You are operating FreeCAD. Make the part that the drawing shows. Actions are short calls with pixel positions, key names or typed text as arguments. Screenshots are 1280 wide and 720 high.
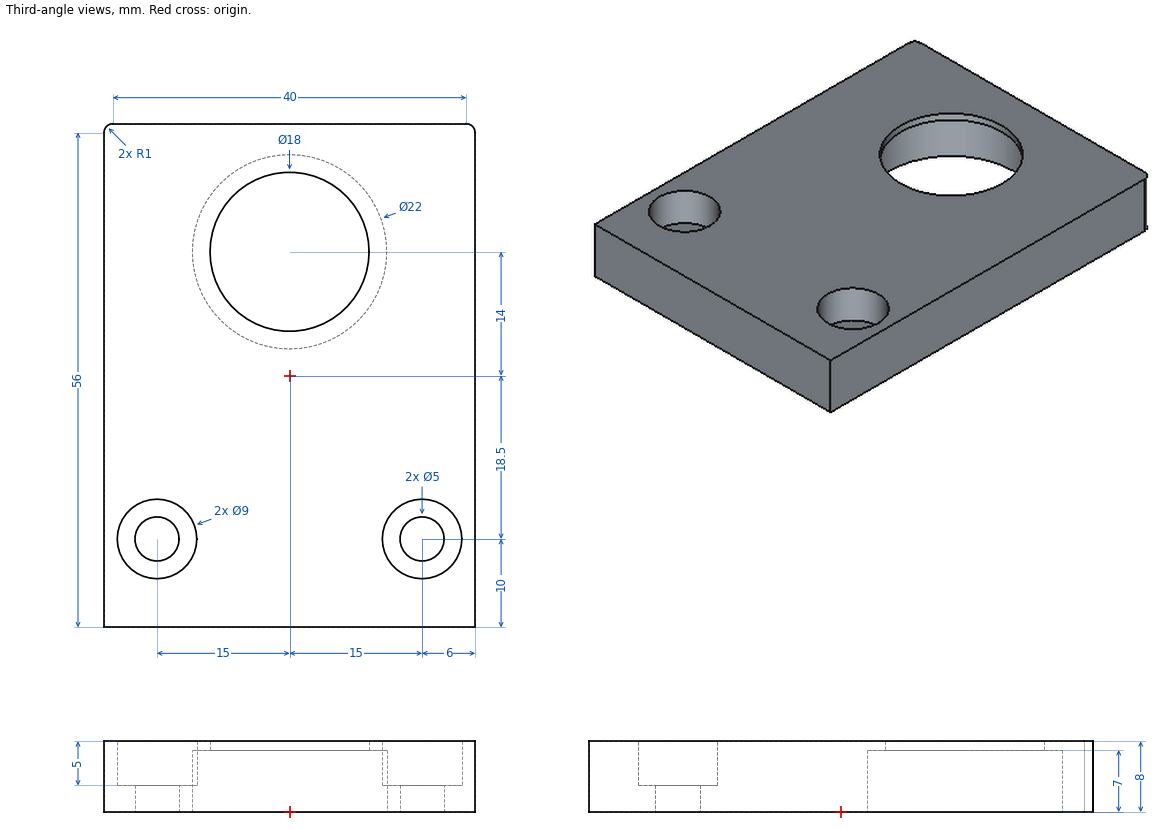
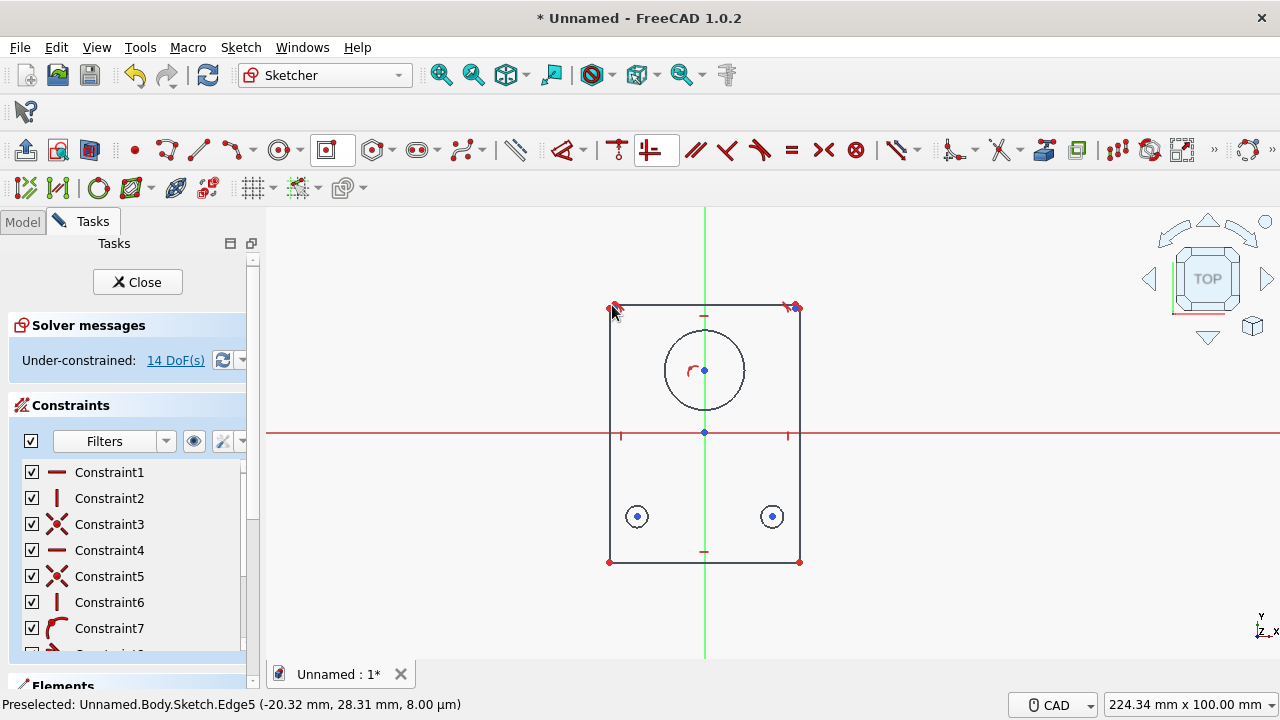
scroll(799, 307, up, 10)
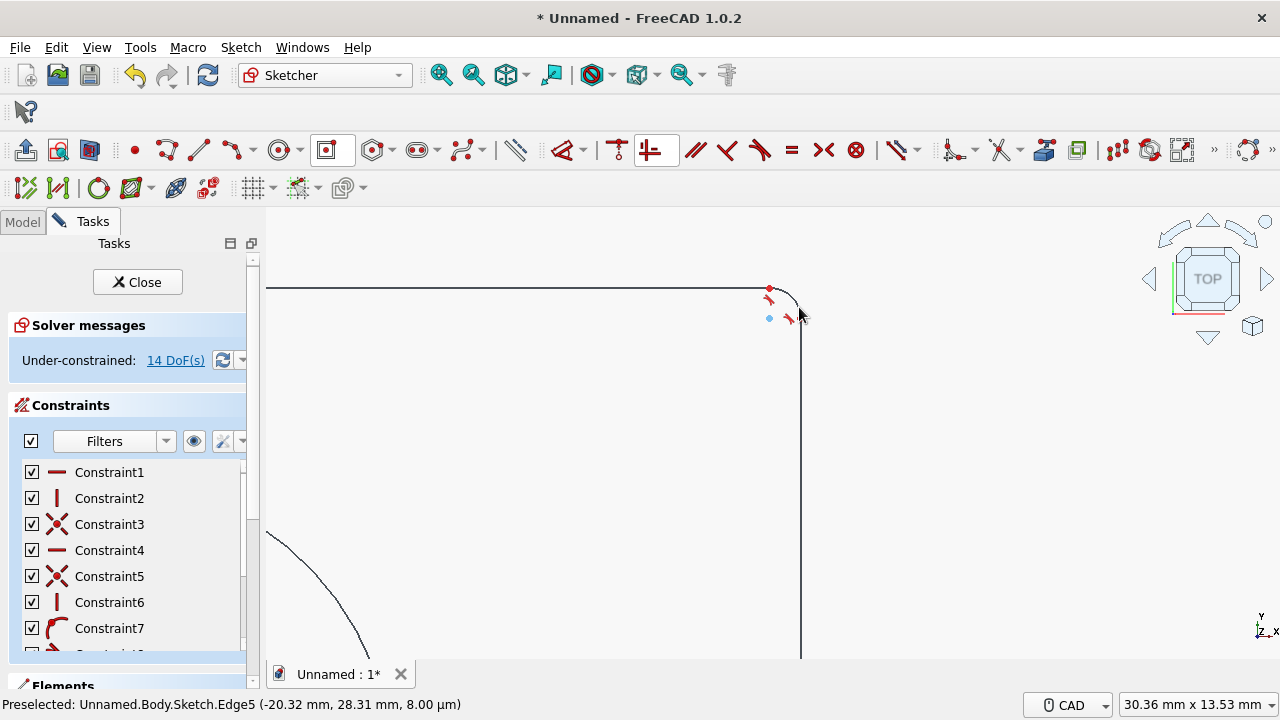
click(798, 305)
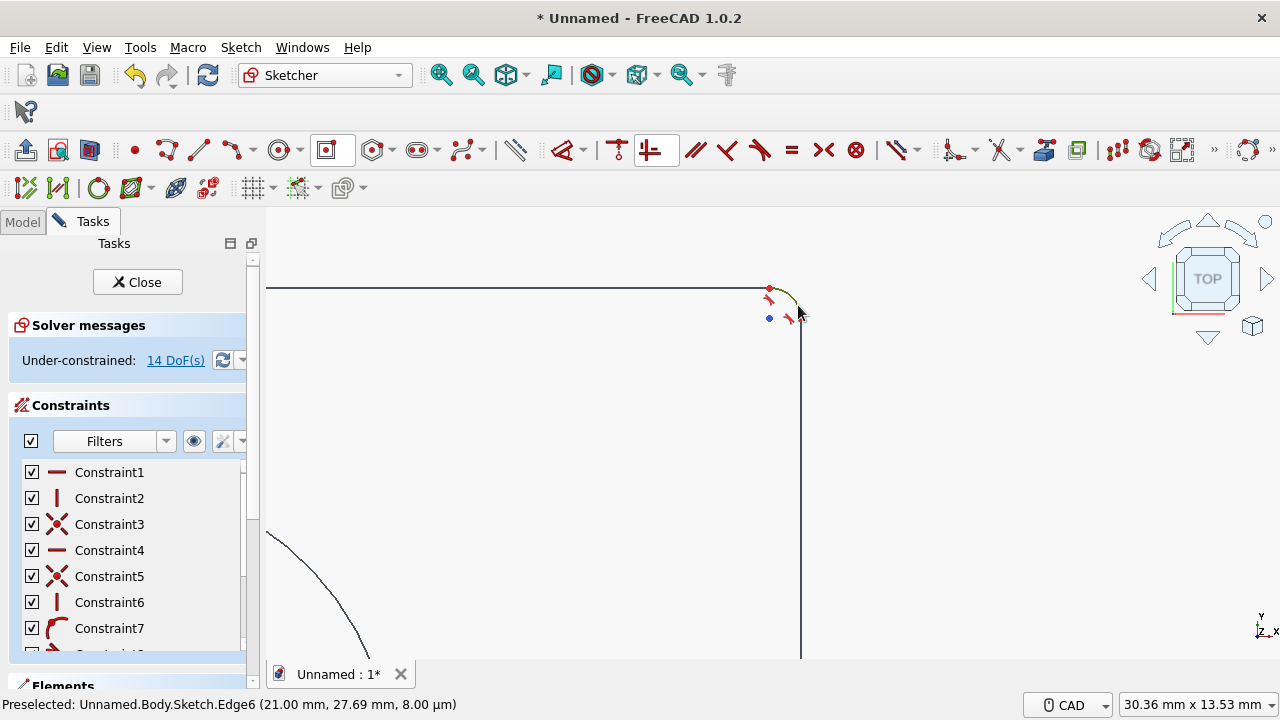
click(792, 150)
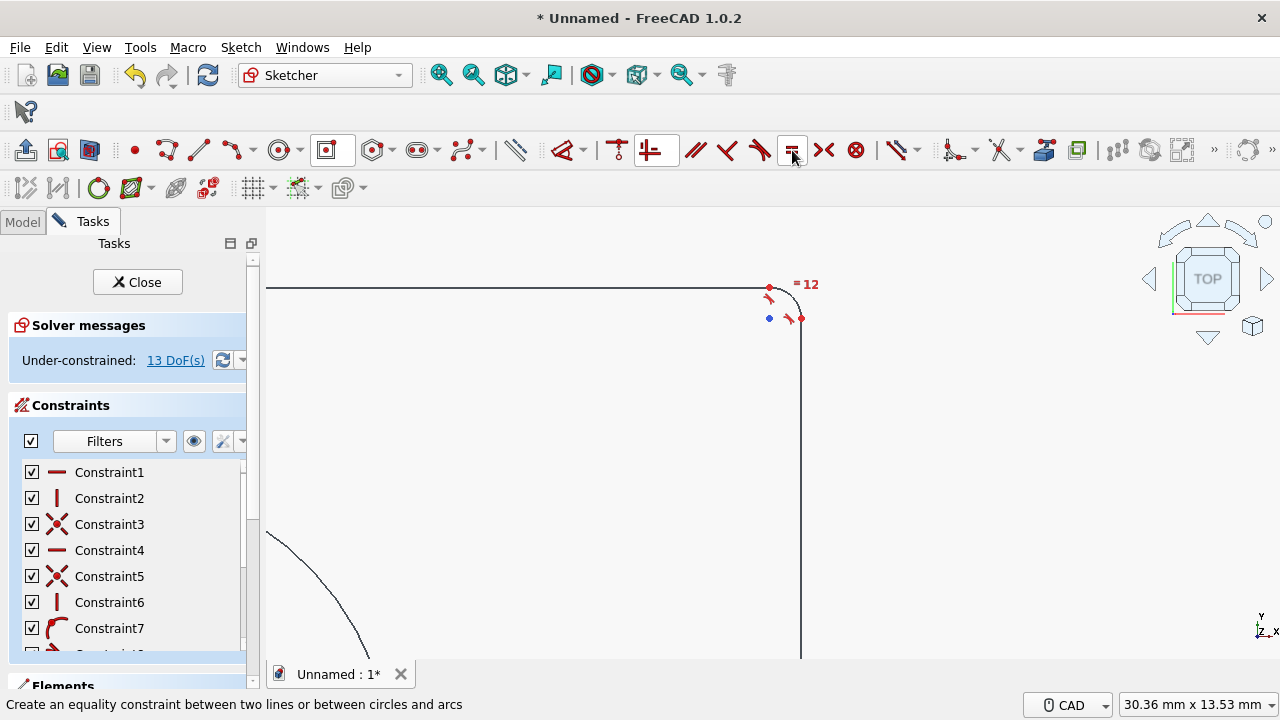
scroll(799, 307, down, 10)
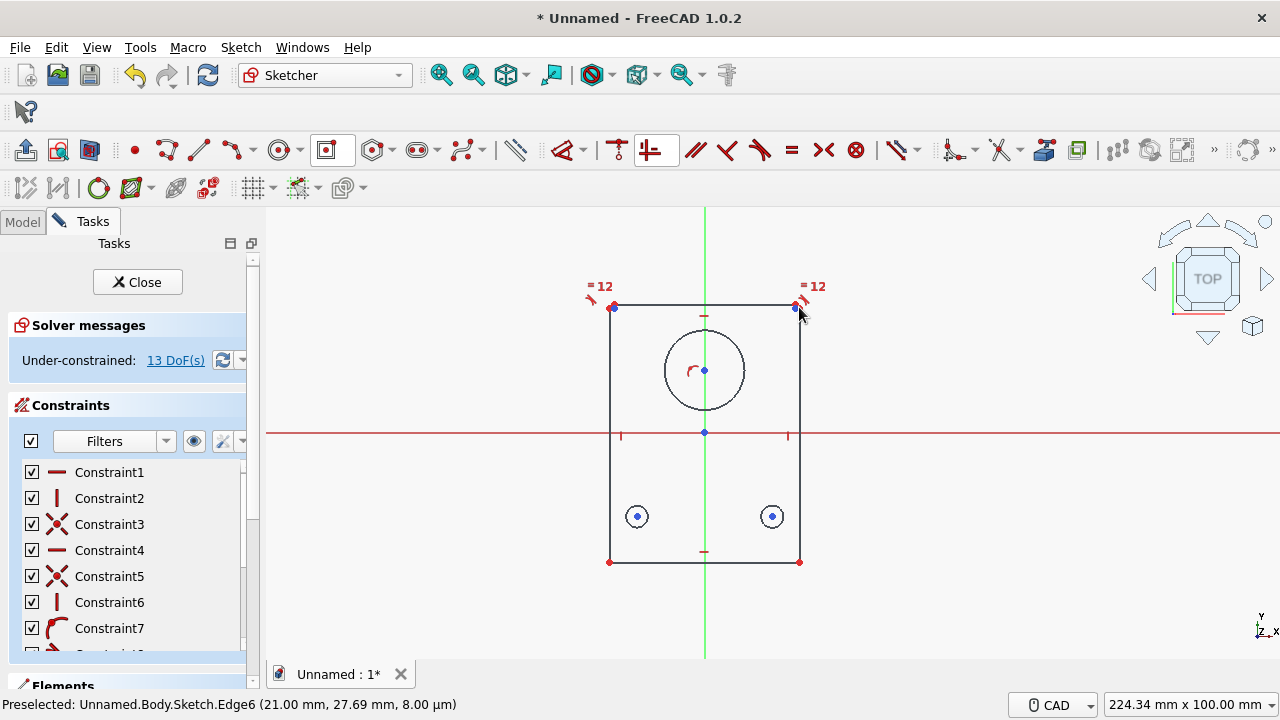
scroll(780, 509, up, 2)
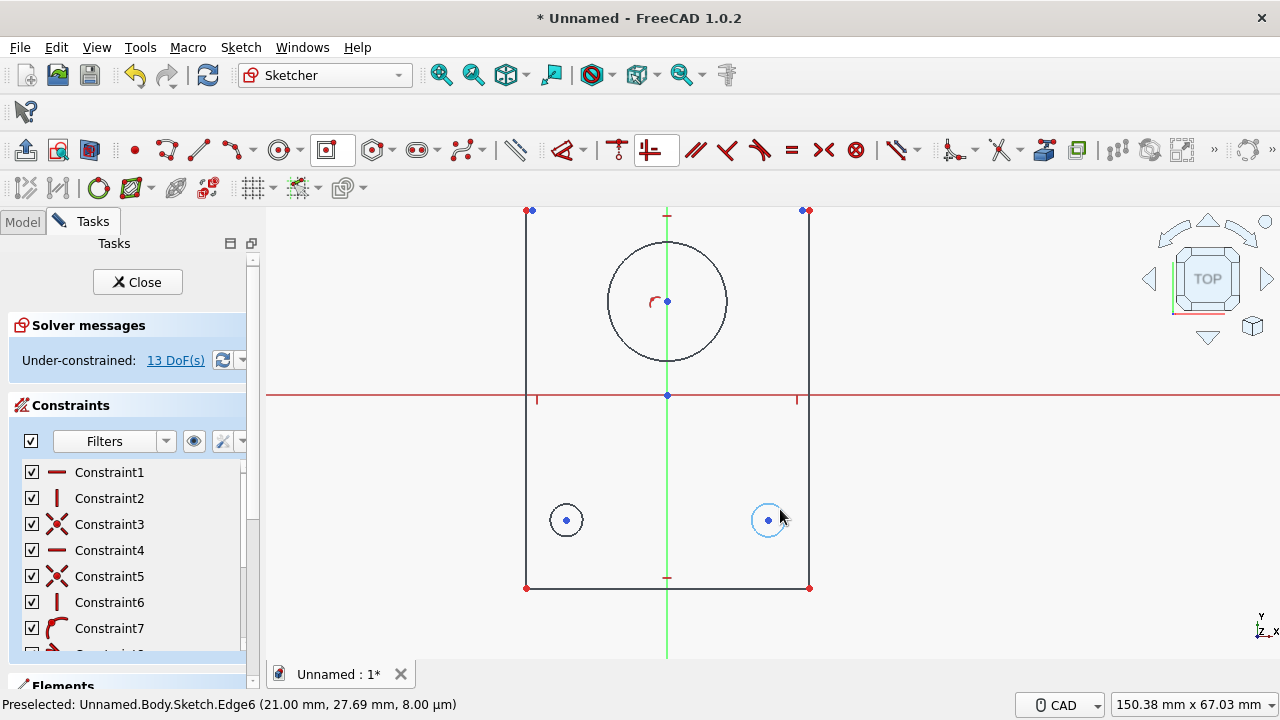
click(780, 508)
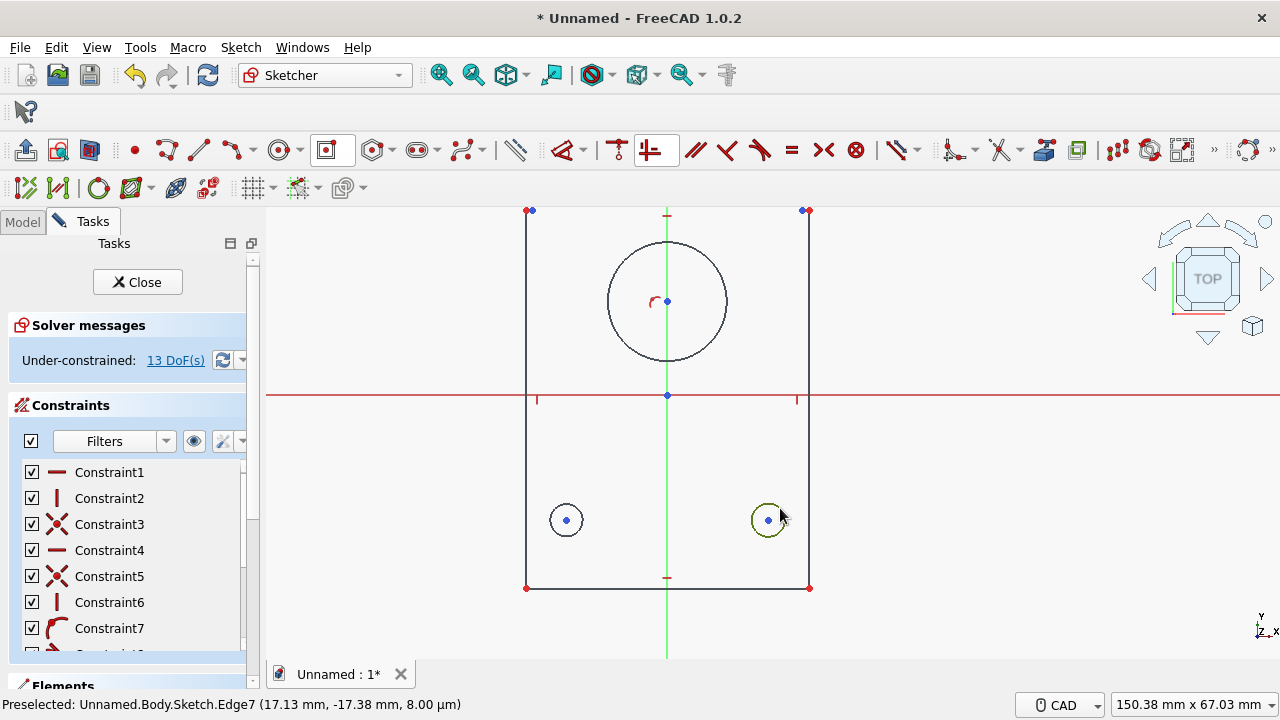
click(578, 509)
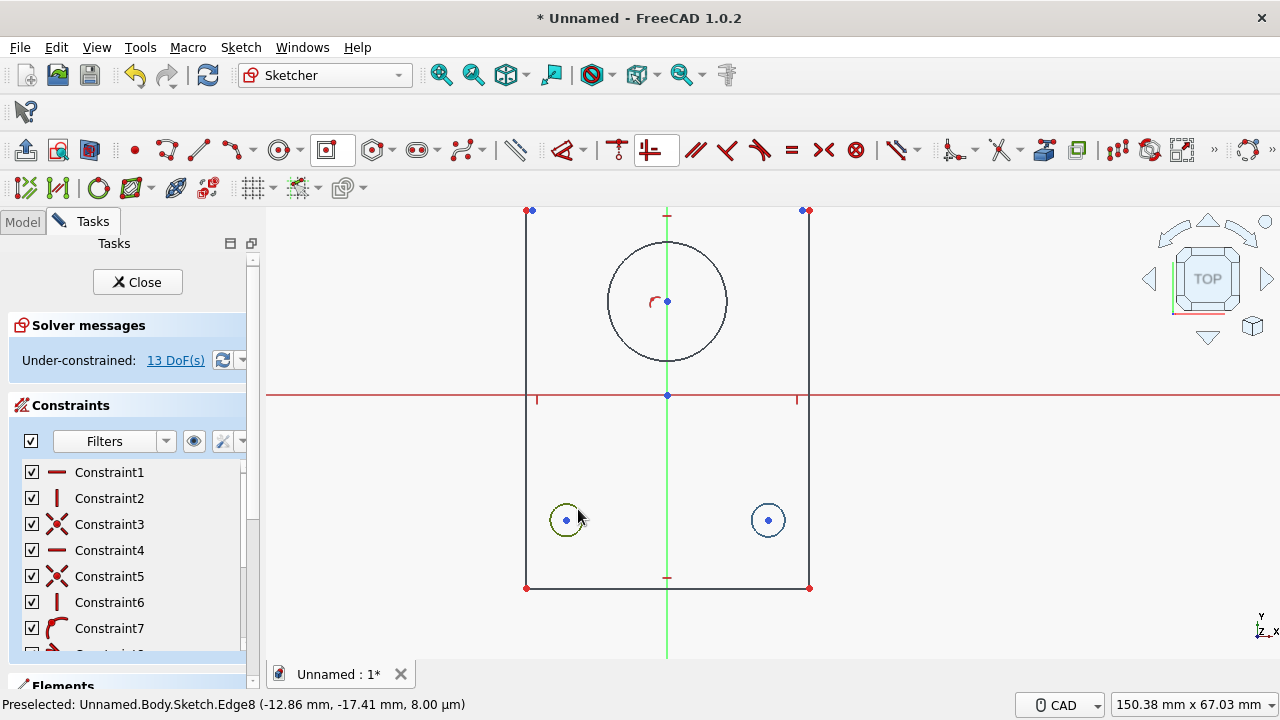
click(792, 150)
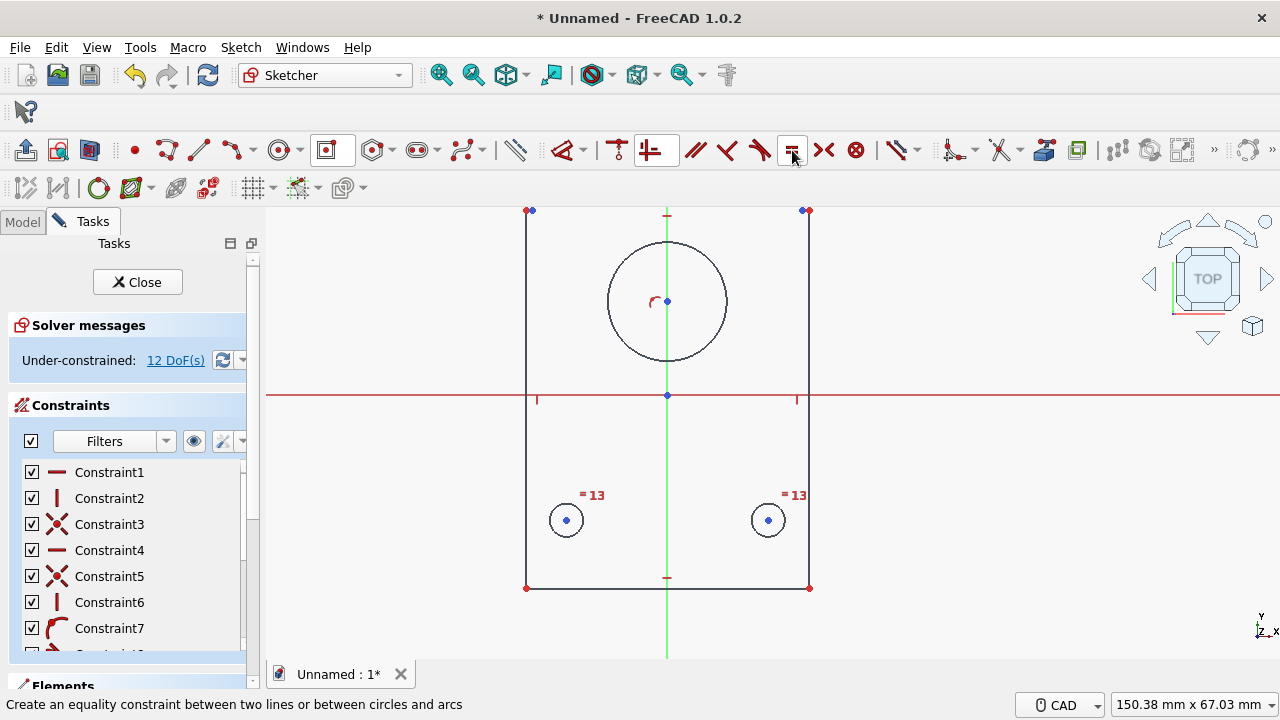
click(768, 520)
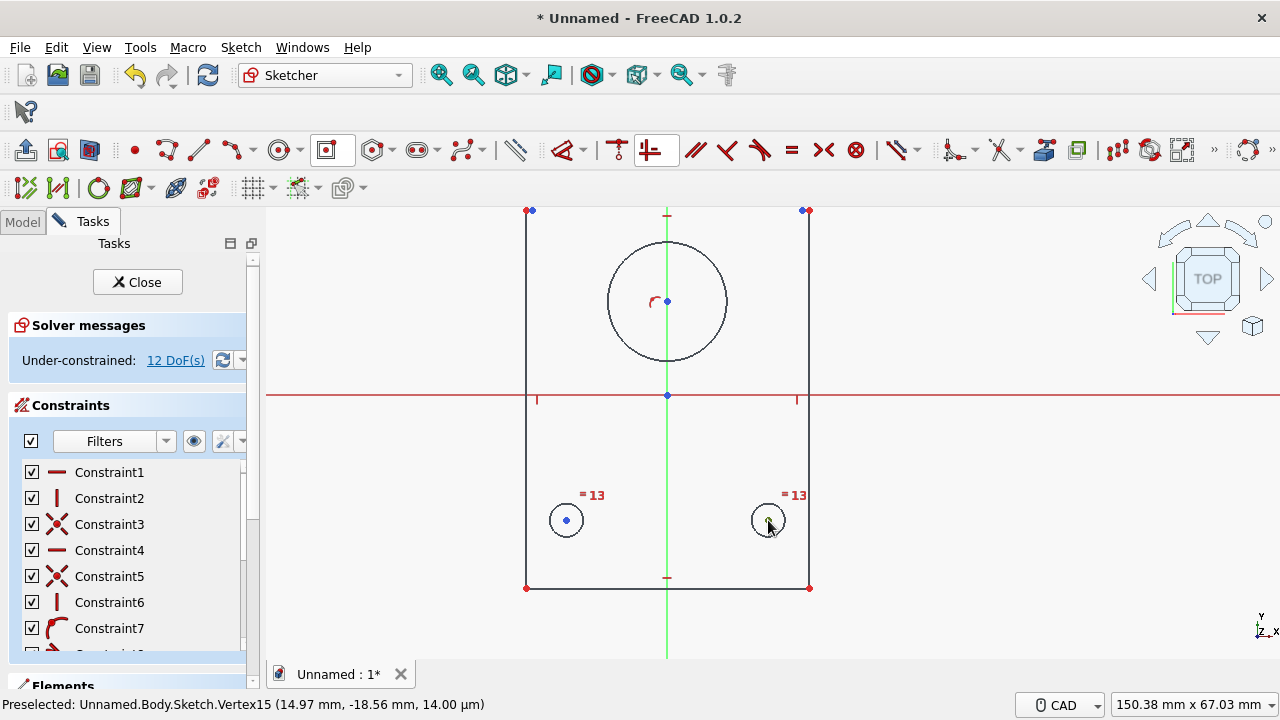
click(566, 520)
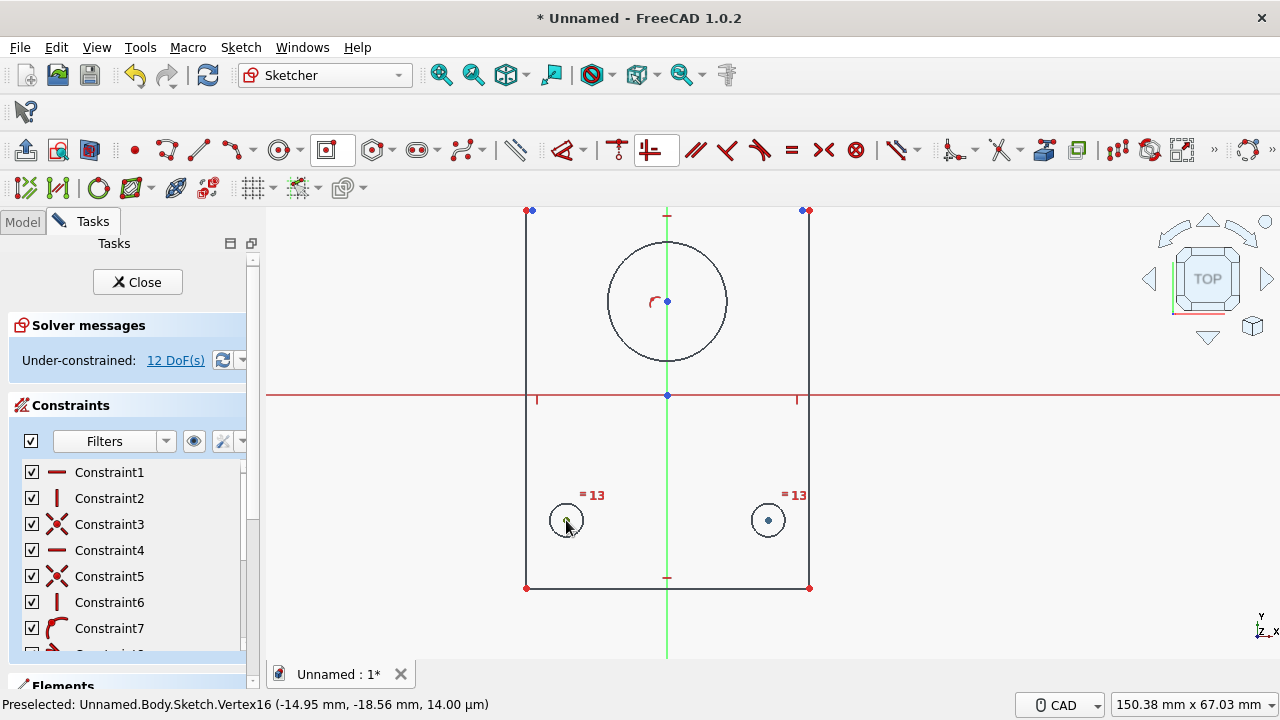
click(674, 150)